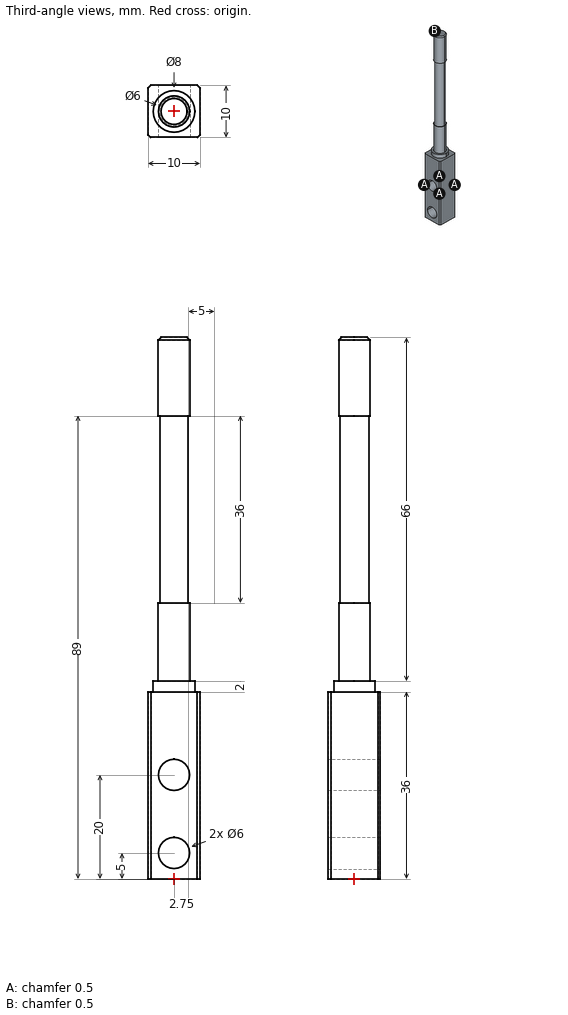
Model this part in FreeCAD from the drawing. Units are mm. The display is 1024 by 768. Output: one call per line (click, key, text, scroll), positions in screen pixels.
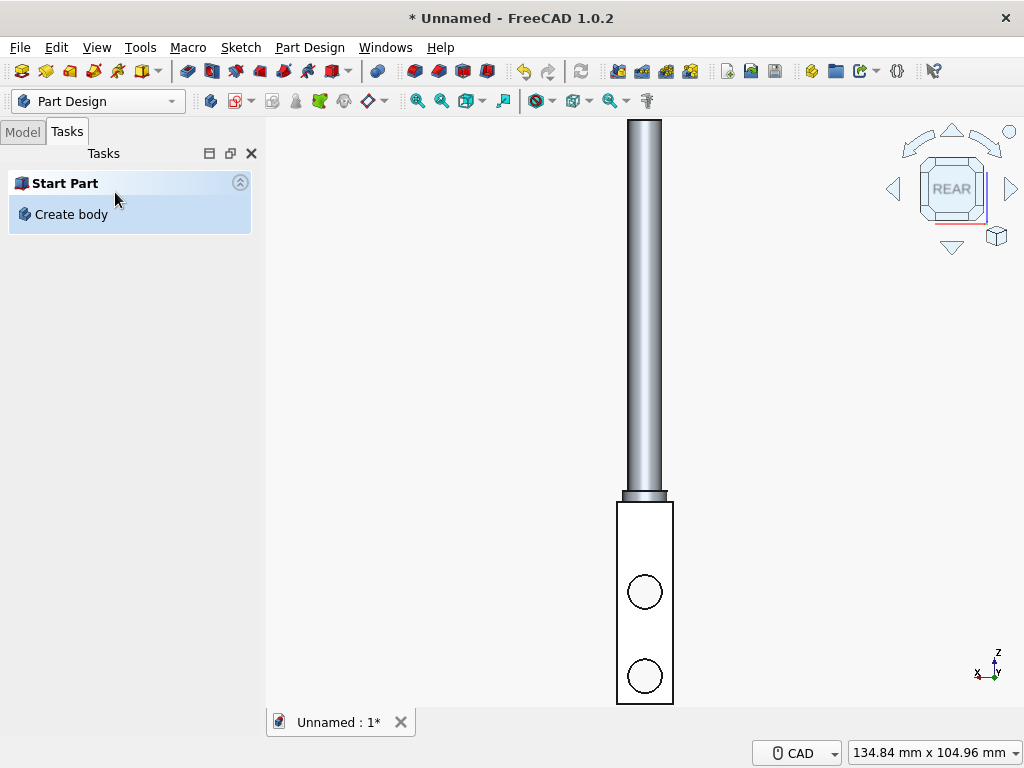
click(673, 602)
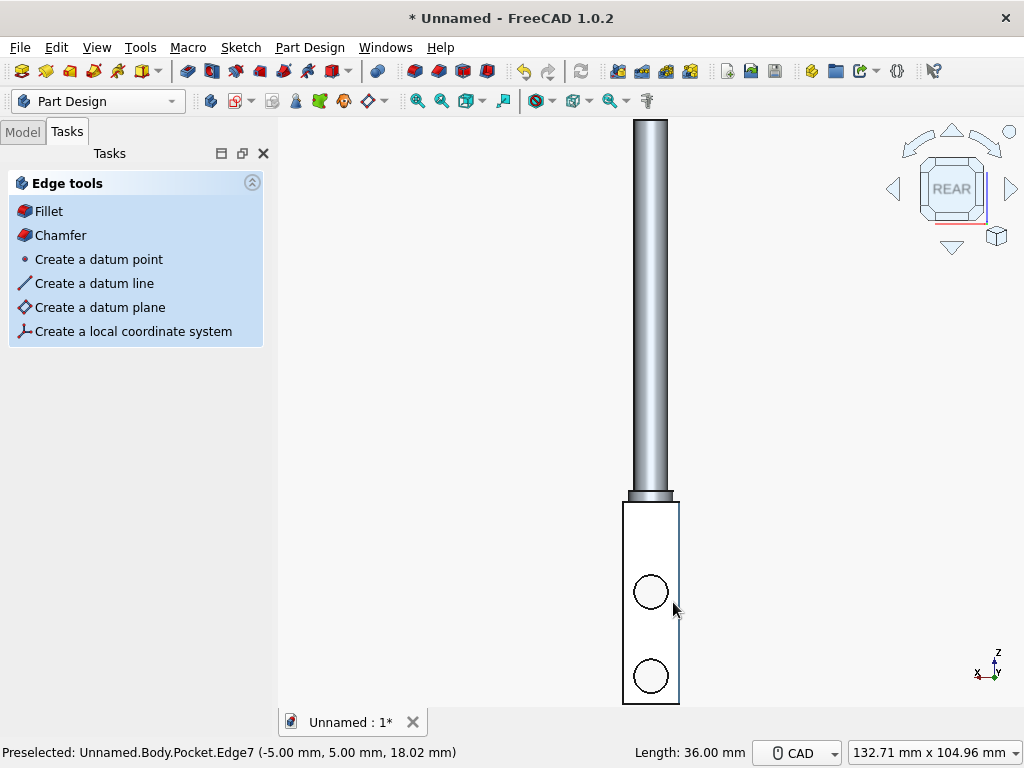
key(0)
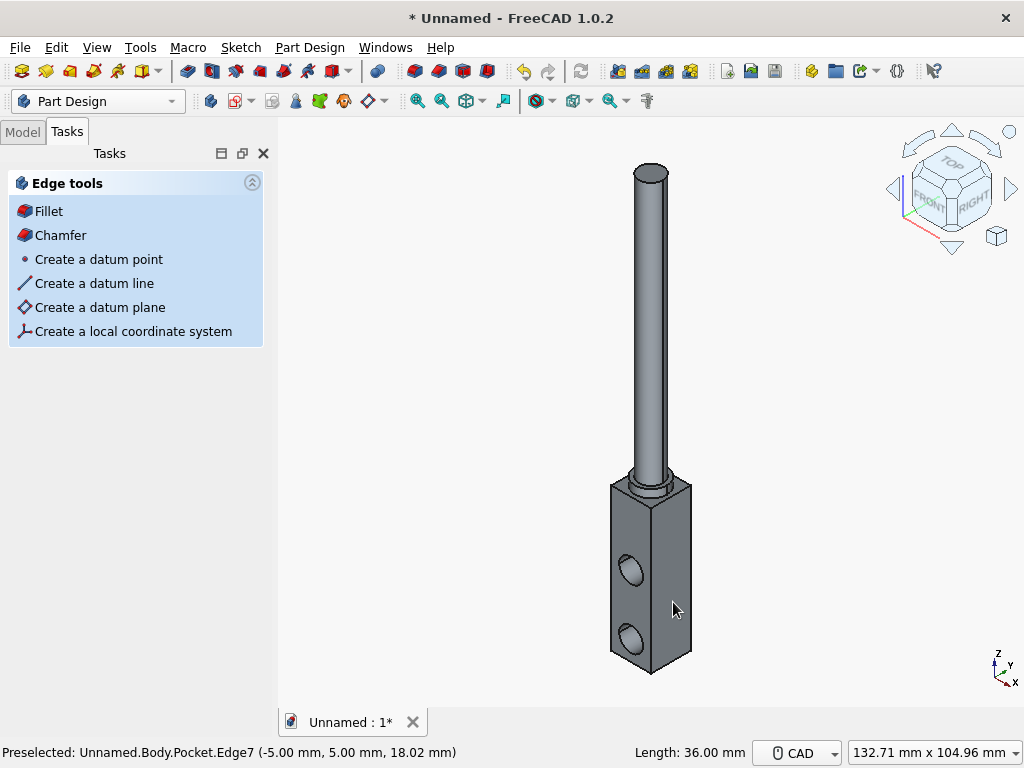
click(651, 590, ctrl)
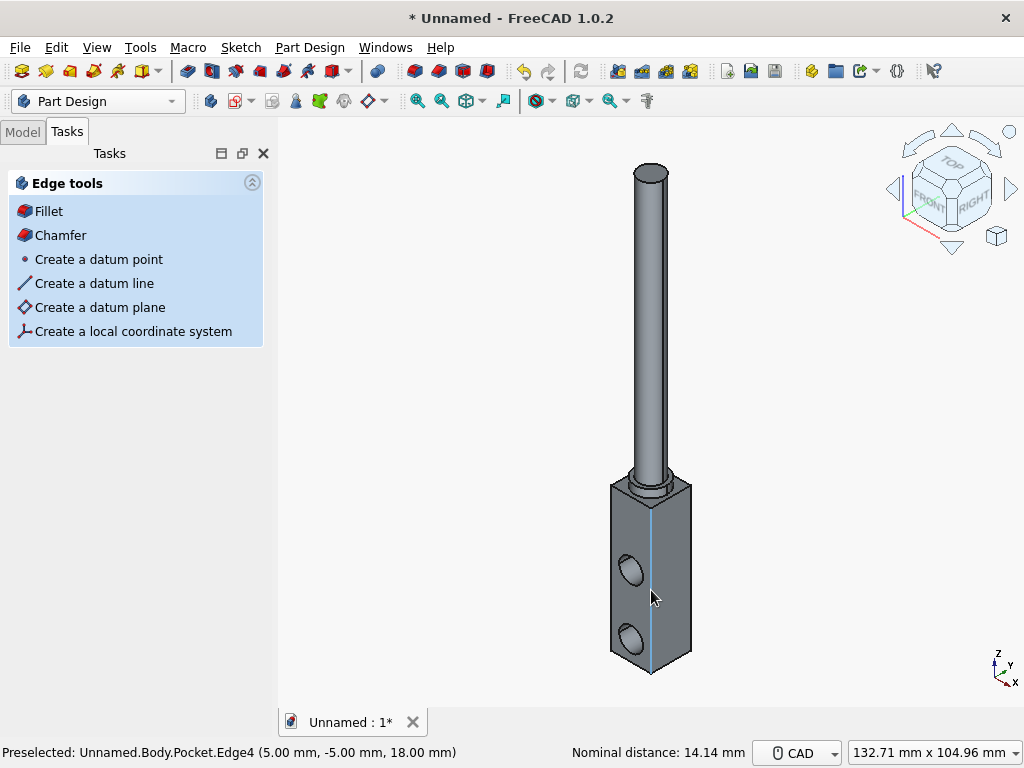
key(2)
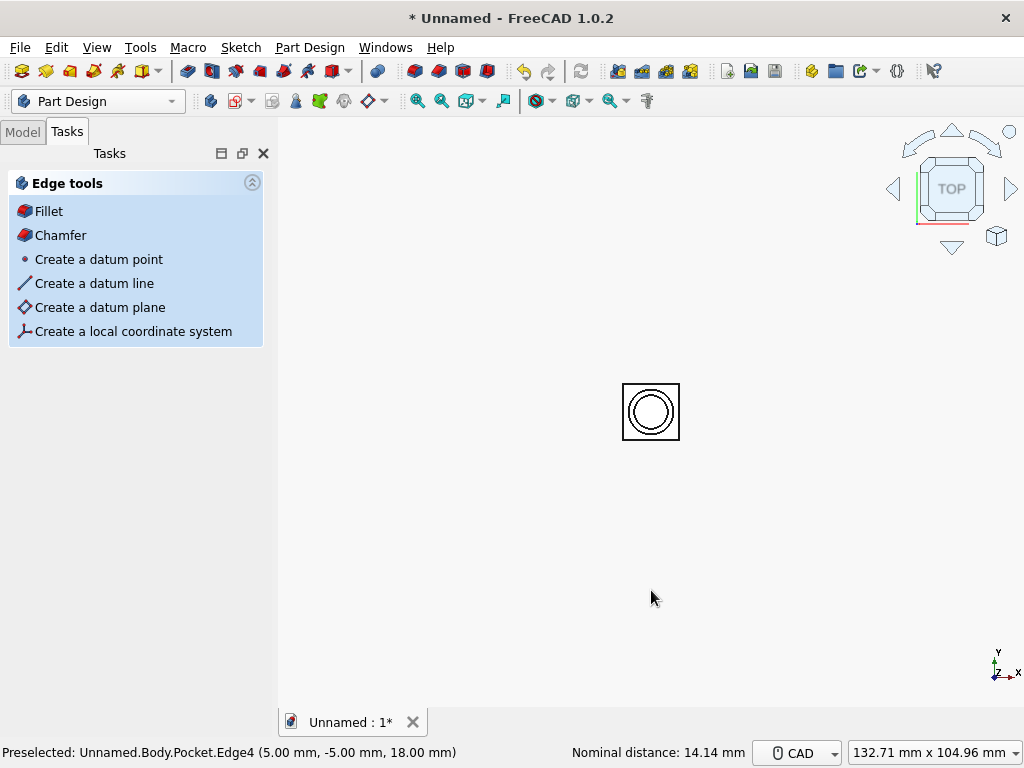
key(v)
key(f)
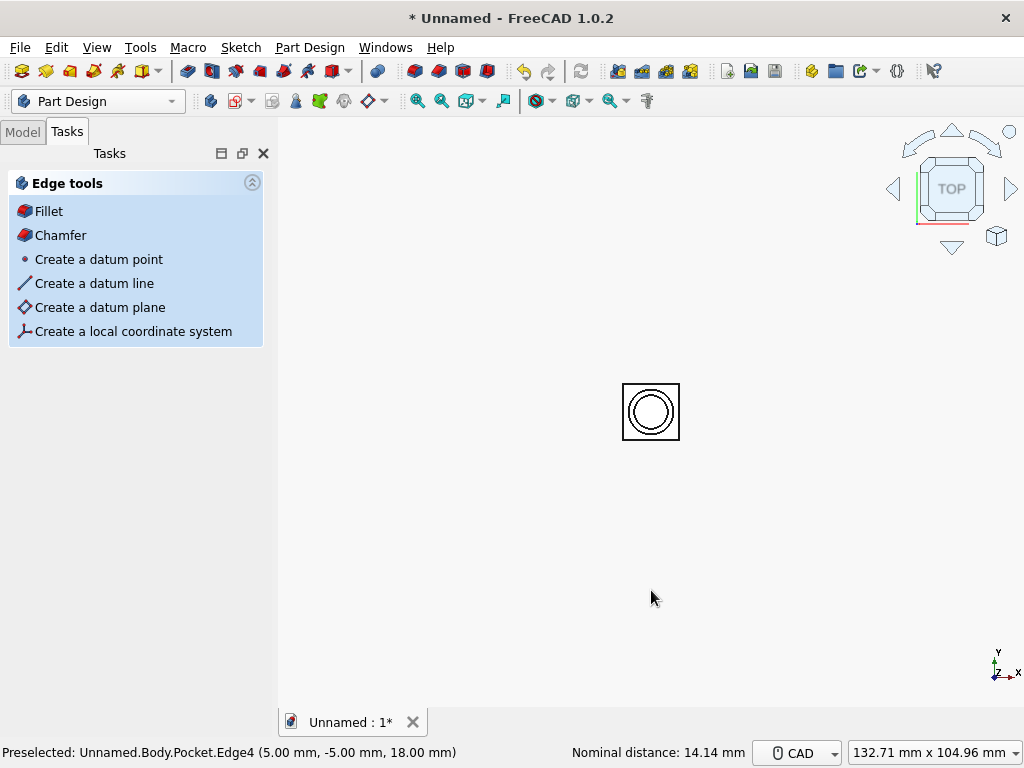
key(1)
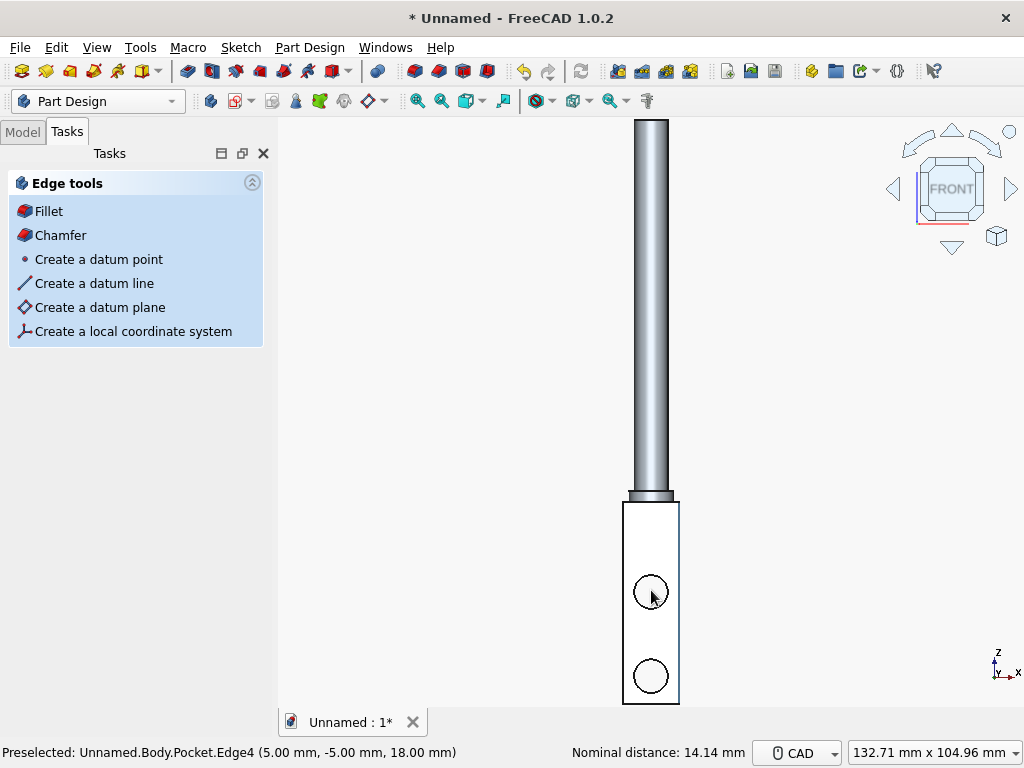
click(623, 602, ctrl)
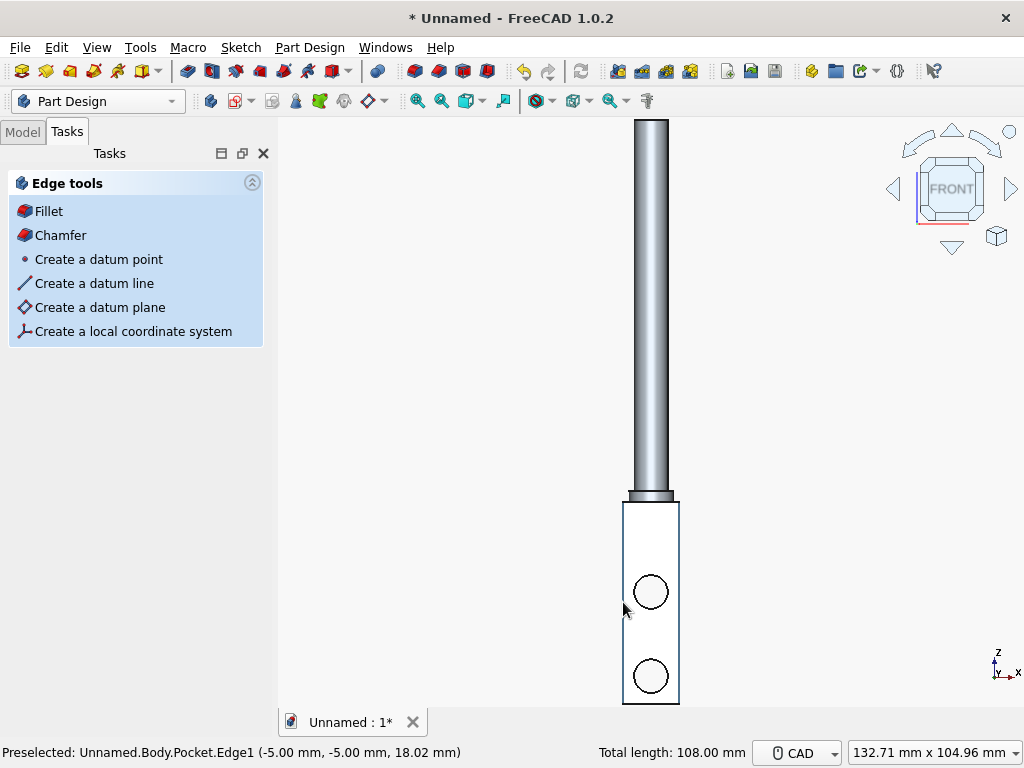
key(3)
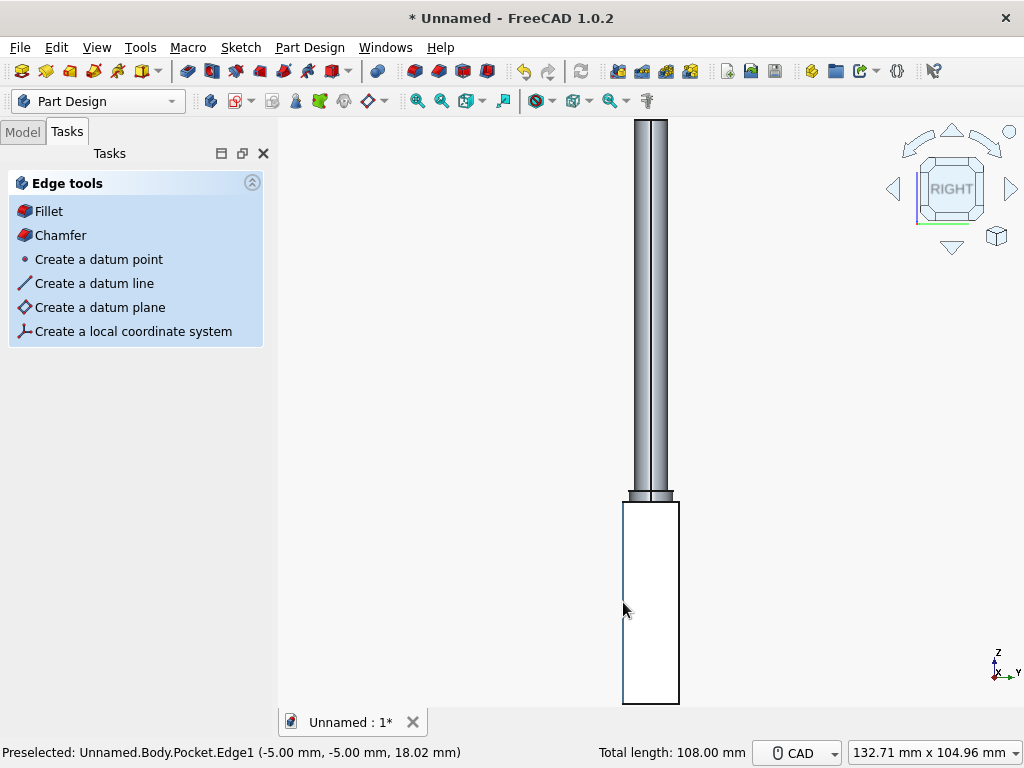
click(679, 602, ctrl)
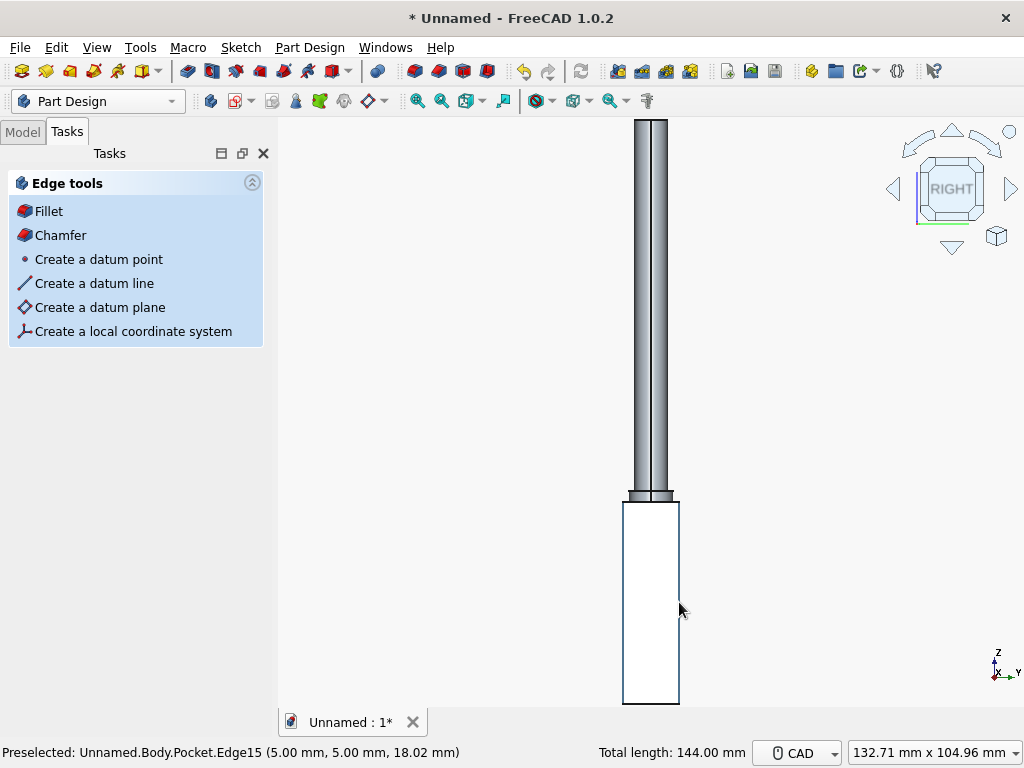
click(440, 72)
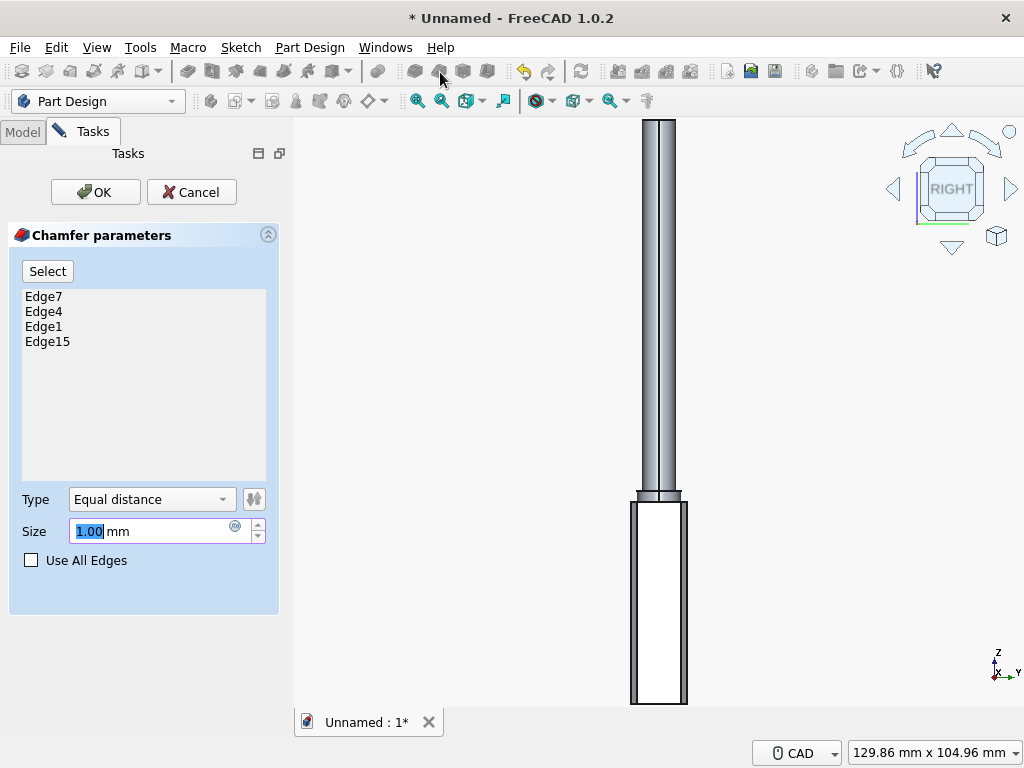
text(0.5)
key(Tab)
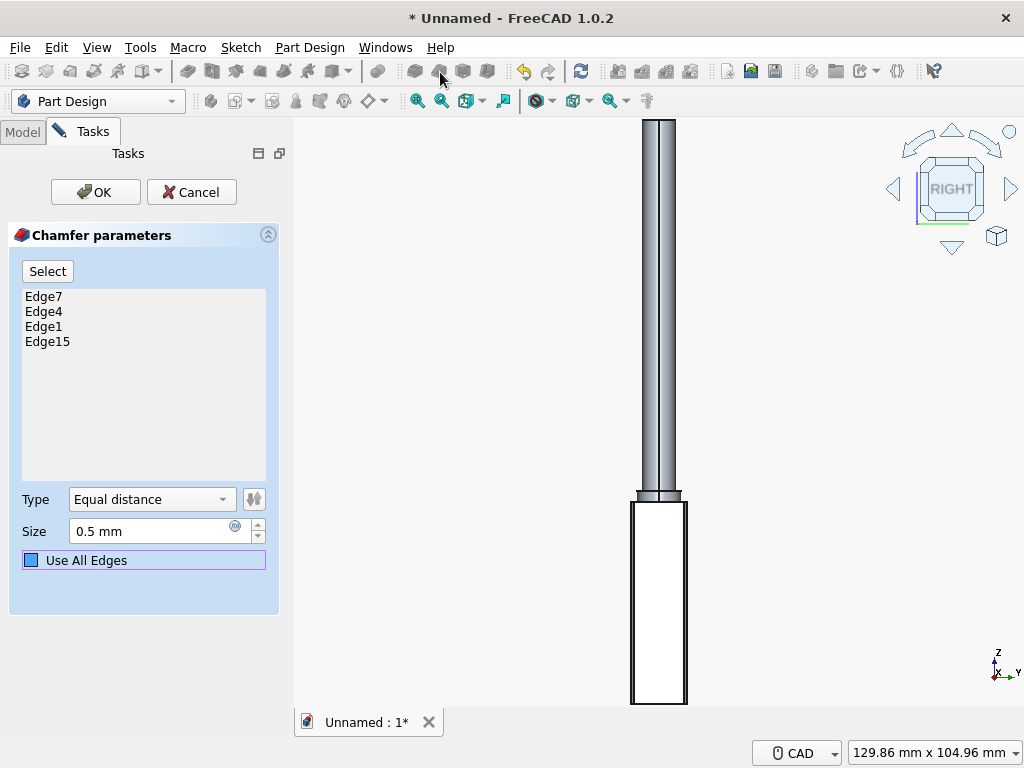
click(96, 192)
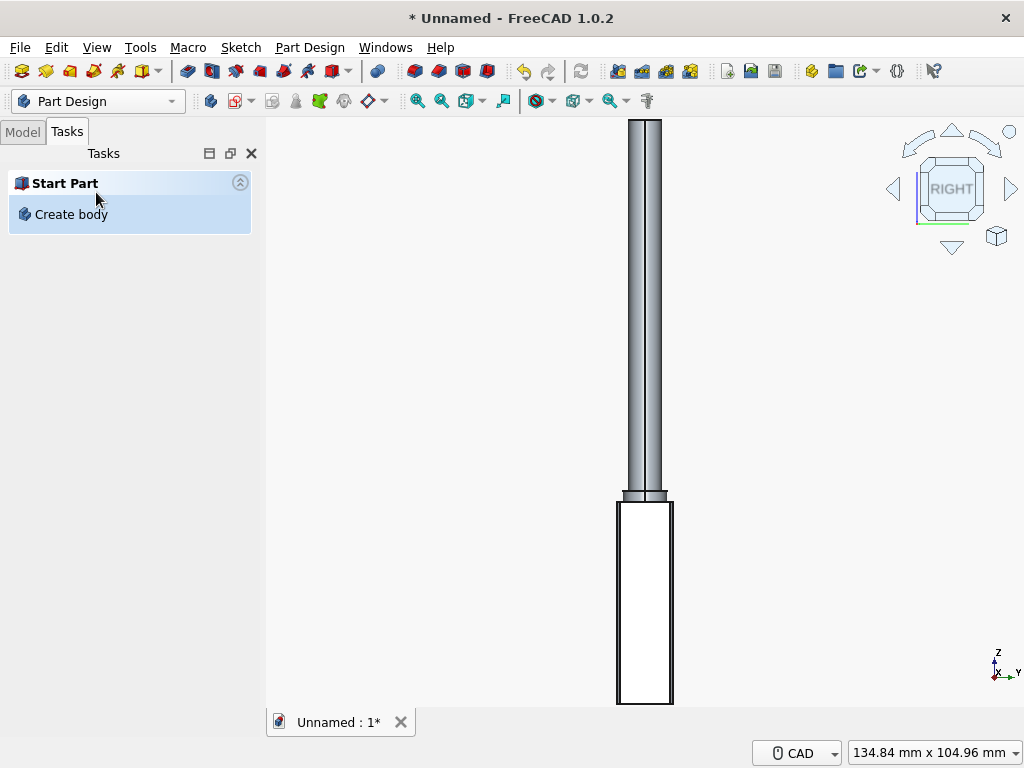
key(0)